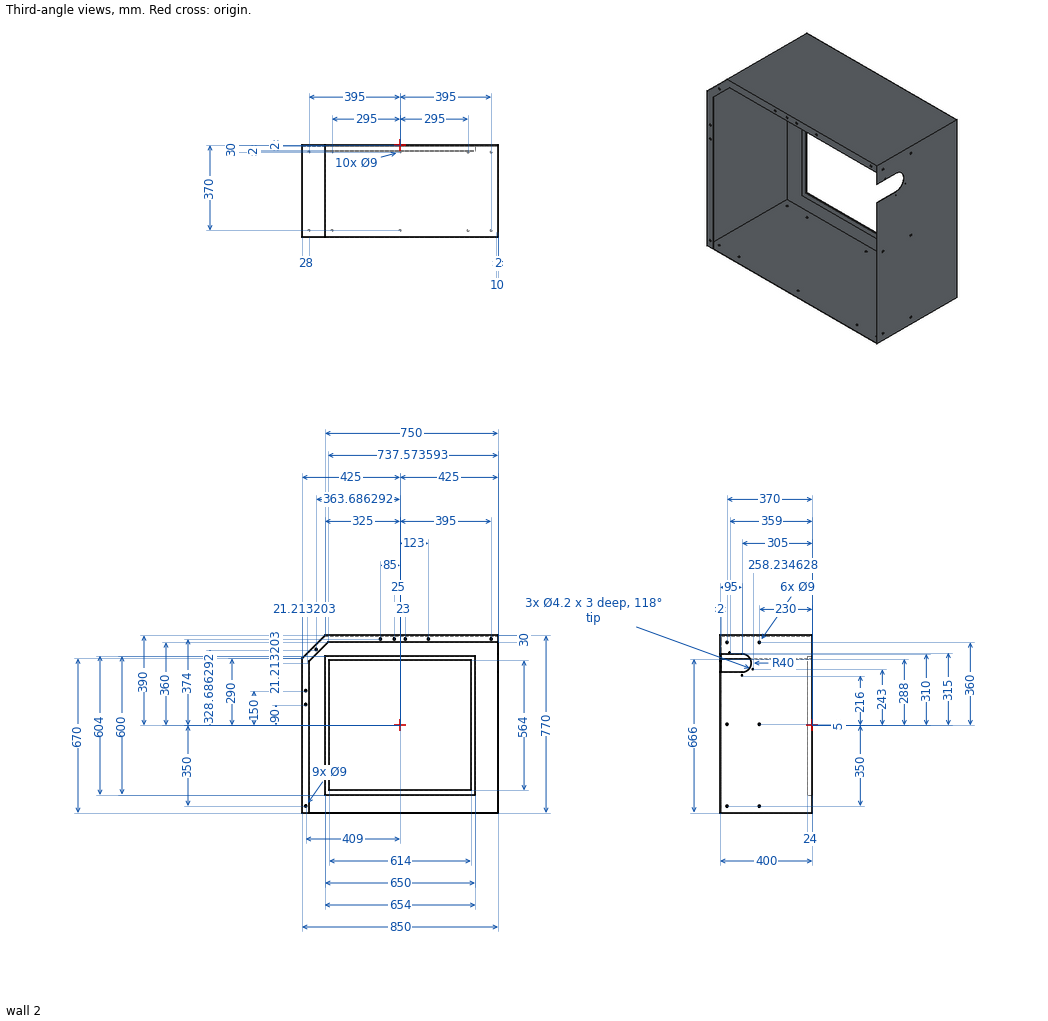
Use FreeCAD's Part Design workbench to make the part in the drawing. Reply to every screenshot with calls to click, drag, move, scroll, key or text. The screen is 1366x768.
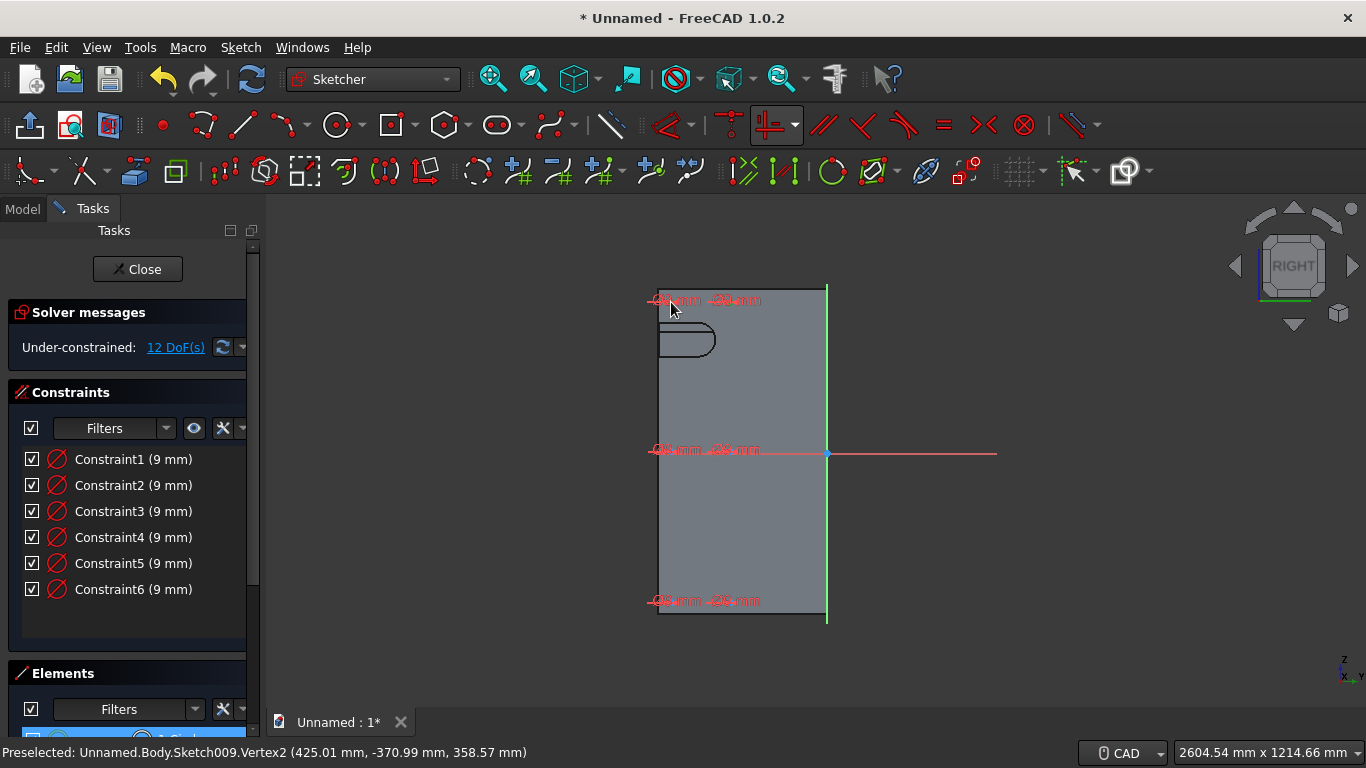
key(h)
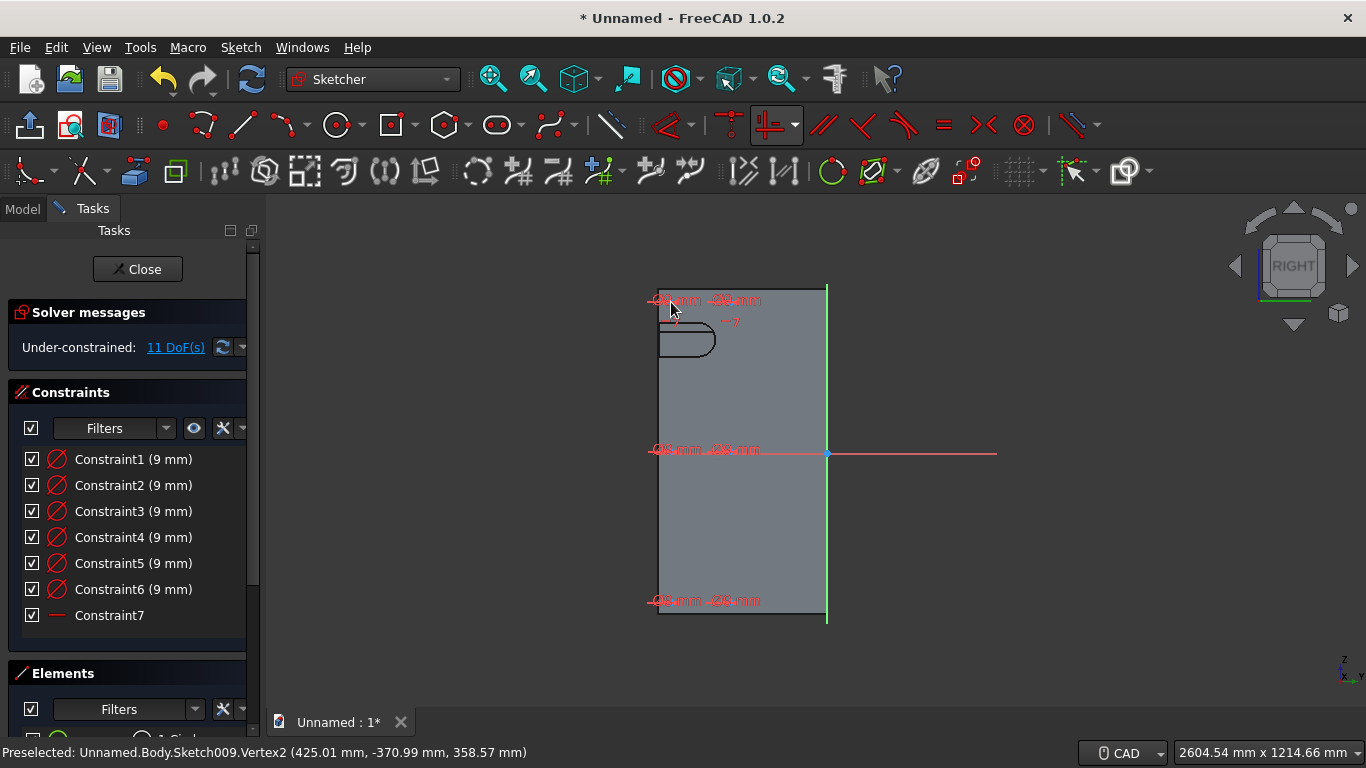
click(731, 302)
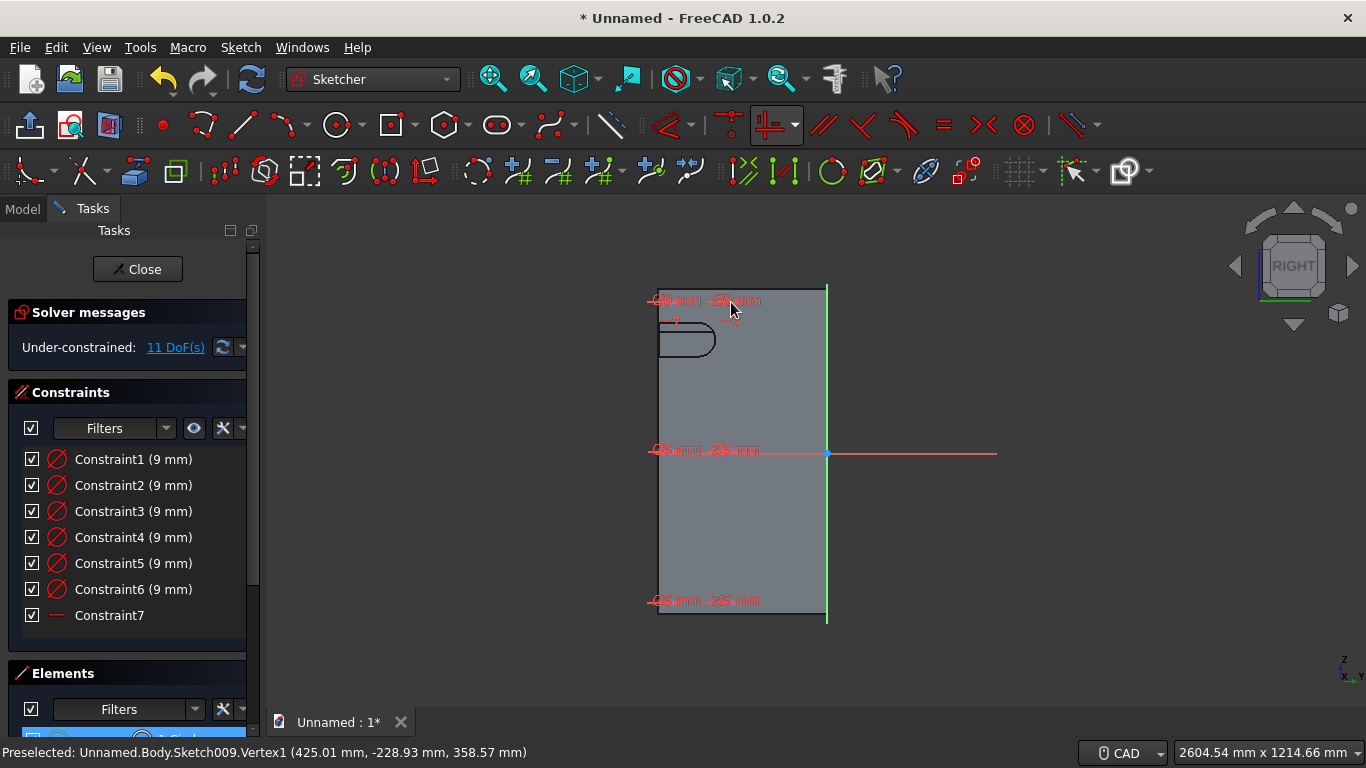
click(730, 452)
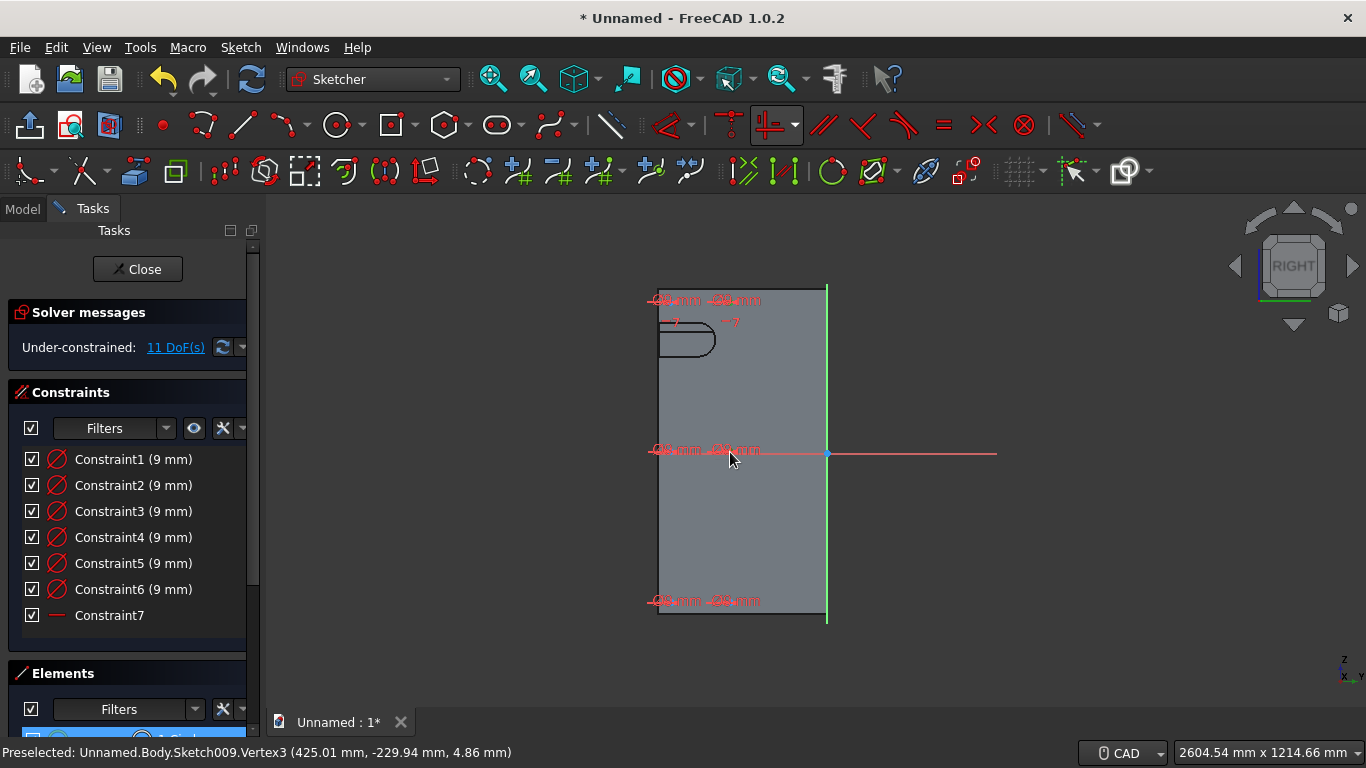
click(798, 126)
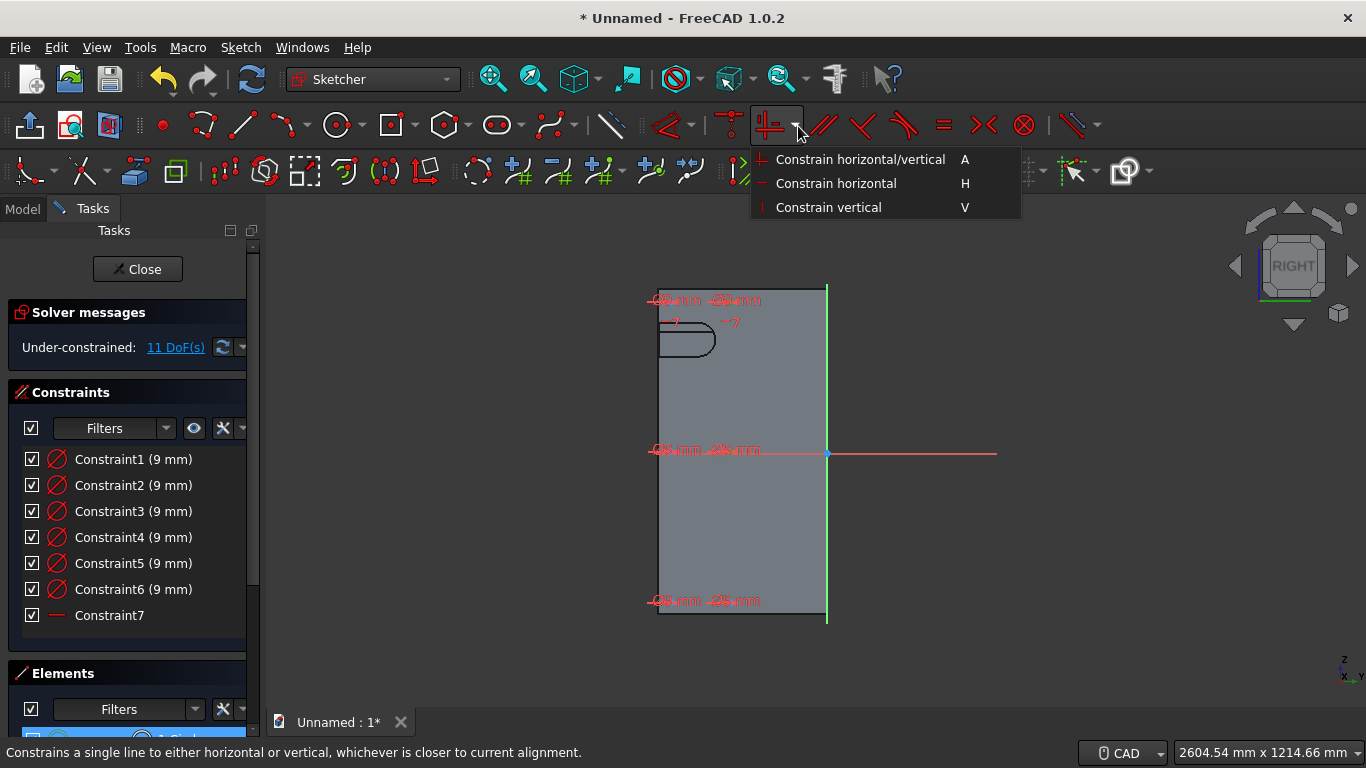
click(886, 207)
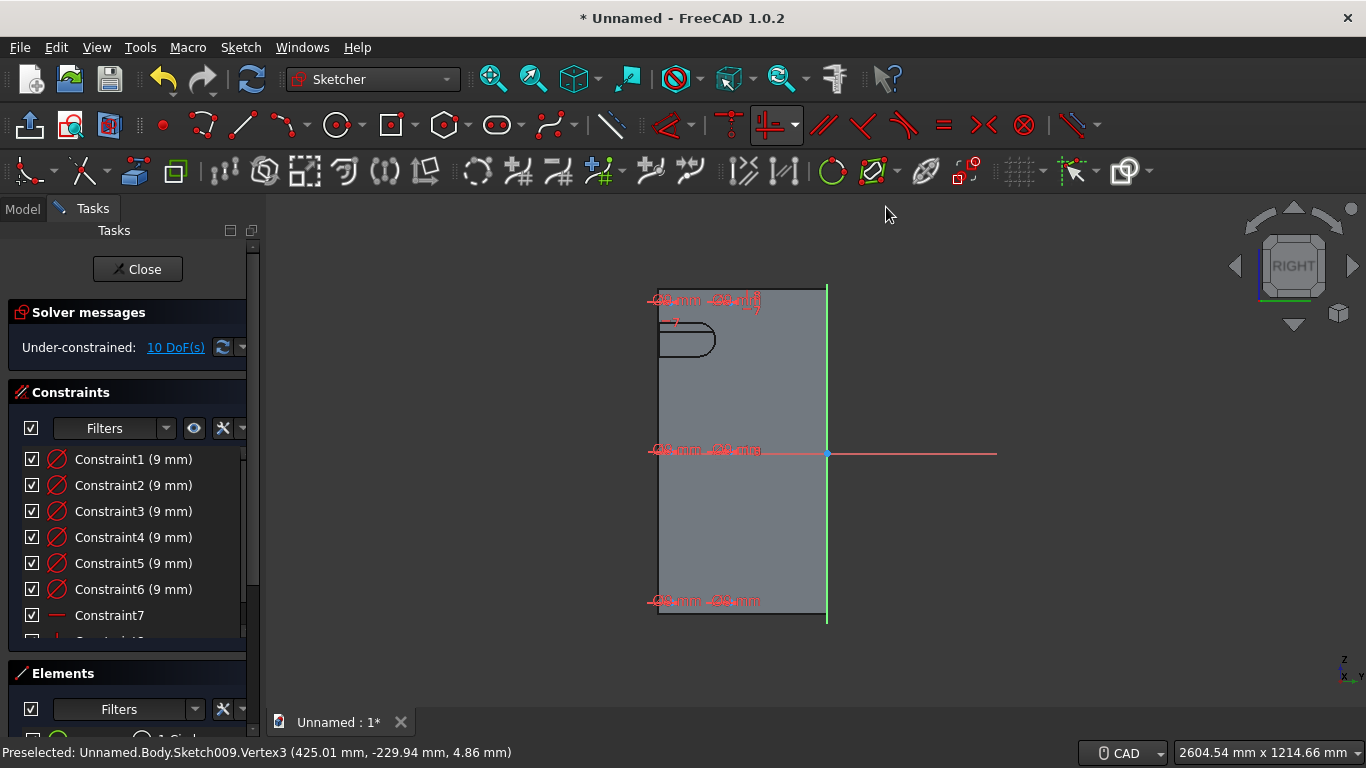
click(671, 302)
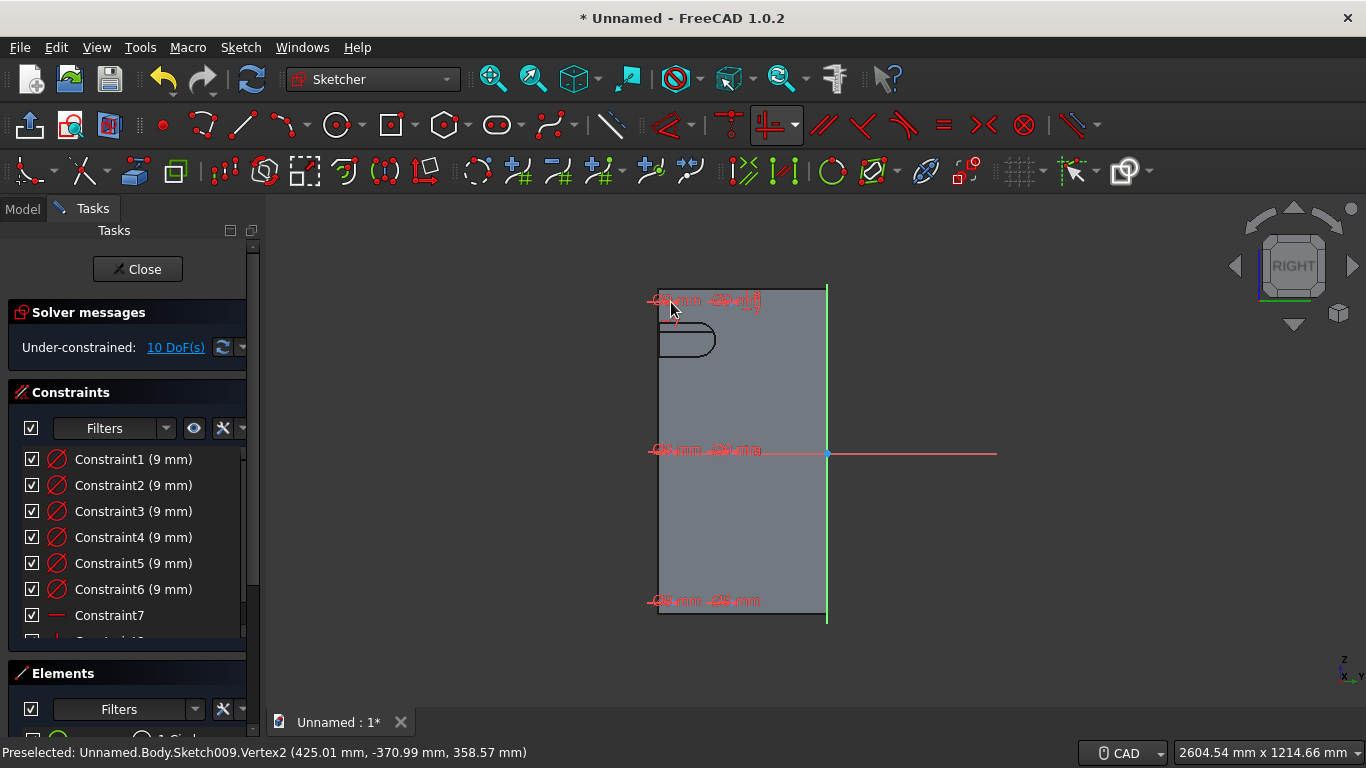
click(671, 452)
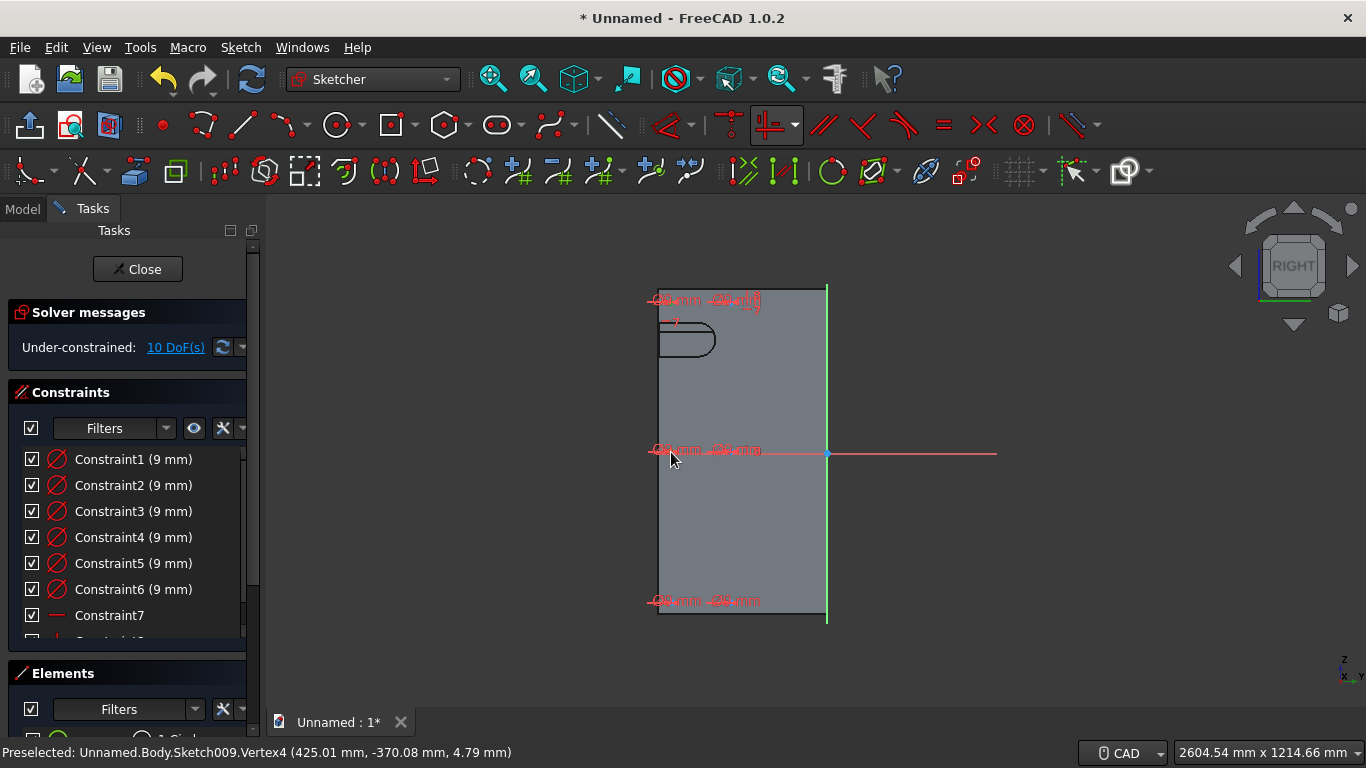
click(798, 126)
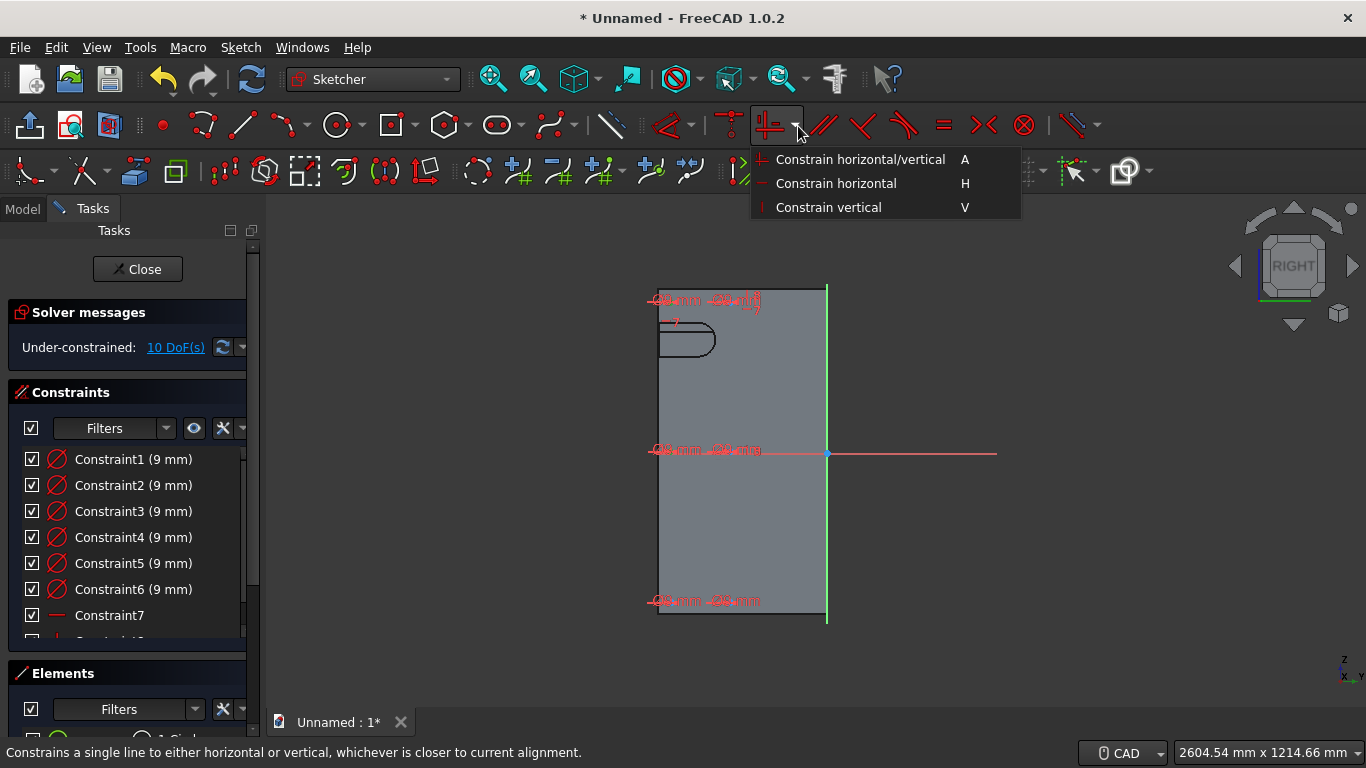
click(886, 207)